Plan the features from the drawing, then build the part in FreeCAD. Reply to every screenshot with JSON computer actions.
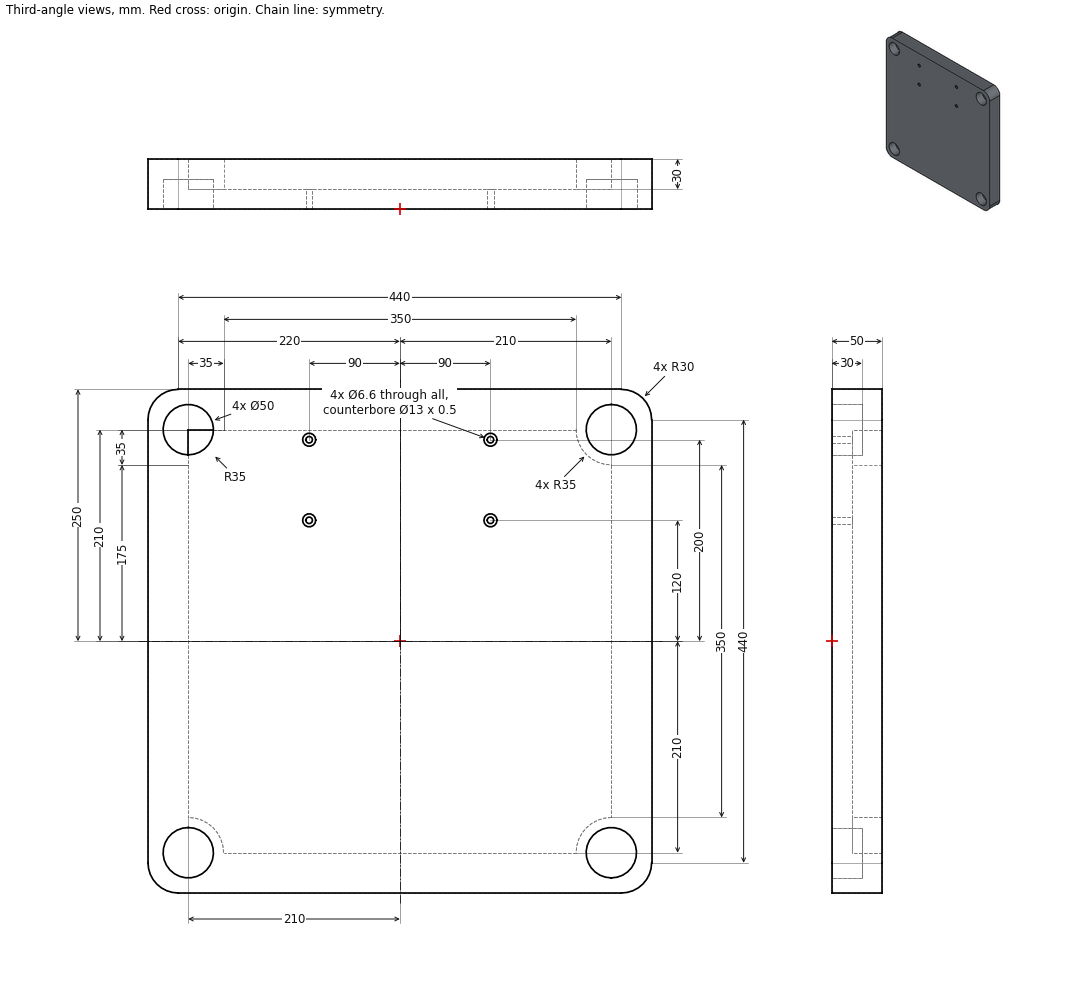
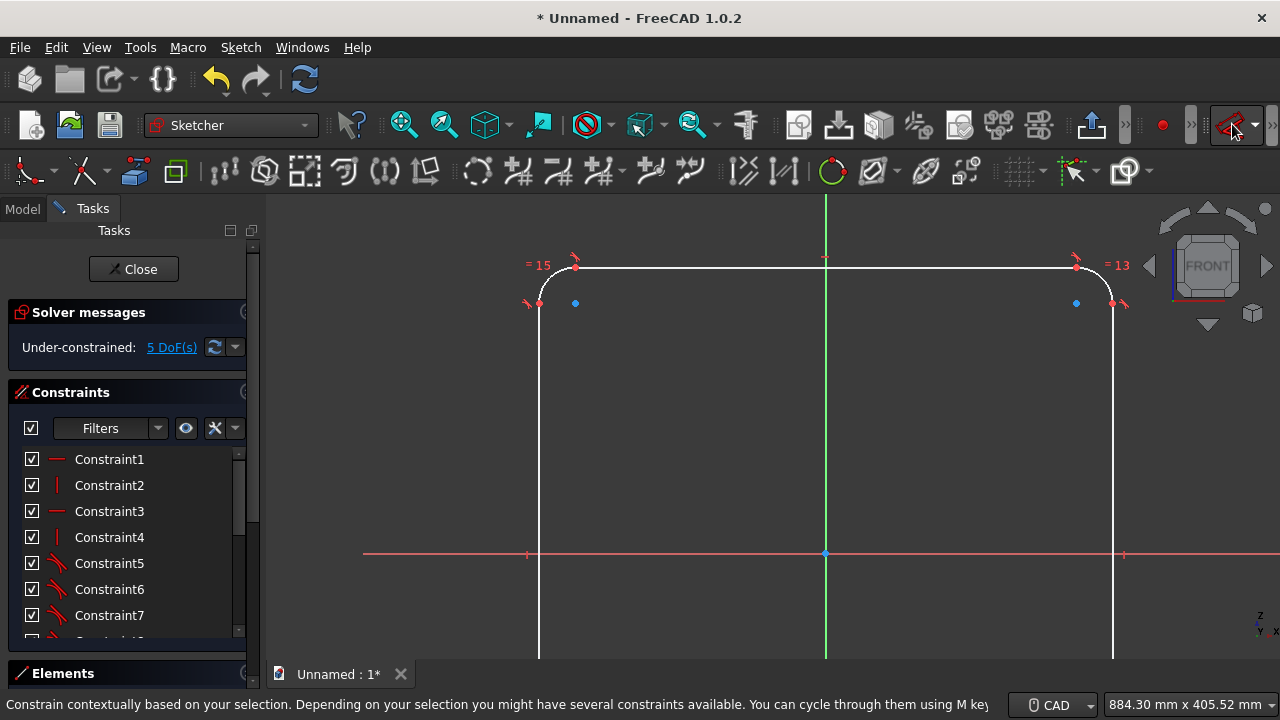
{"action": "left_click", "coordinate": [1109, 287]}
{"action": "left_click", "coordinate": [1083, 235]}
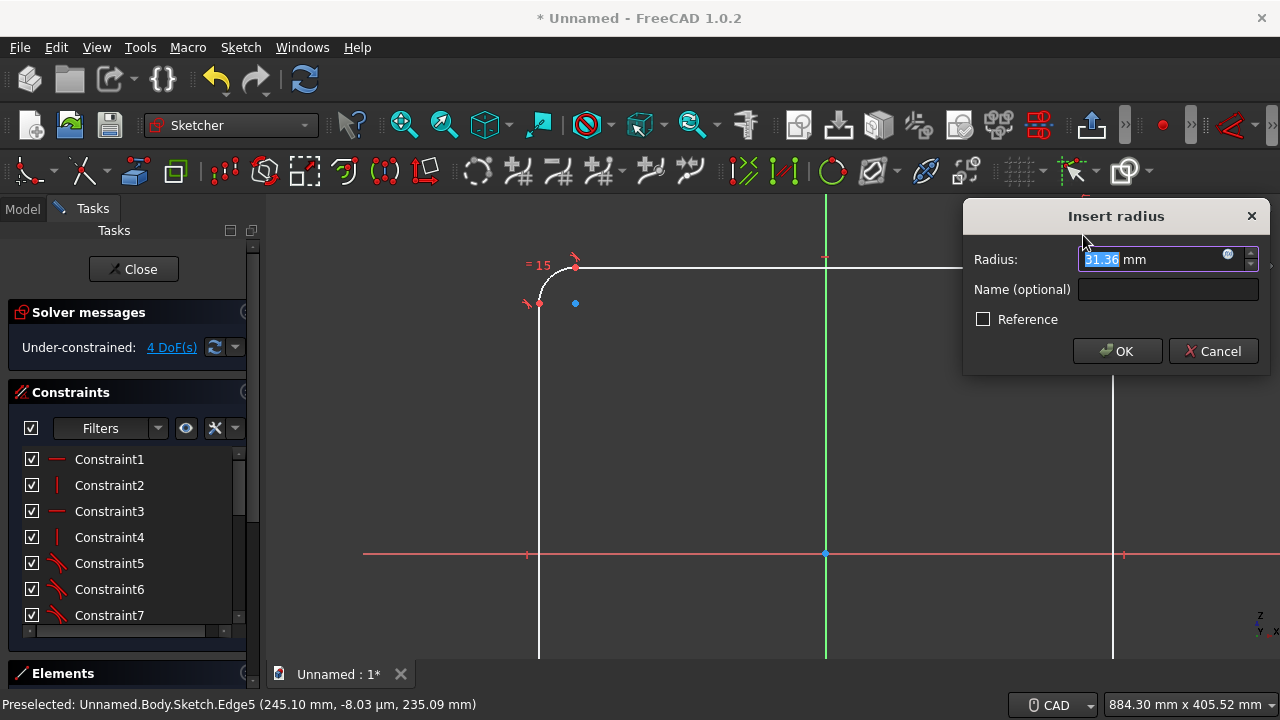
{"action": "type", "text": "30"}
{"action": "key", "text": "Return"}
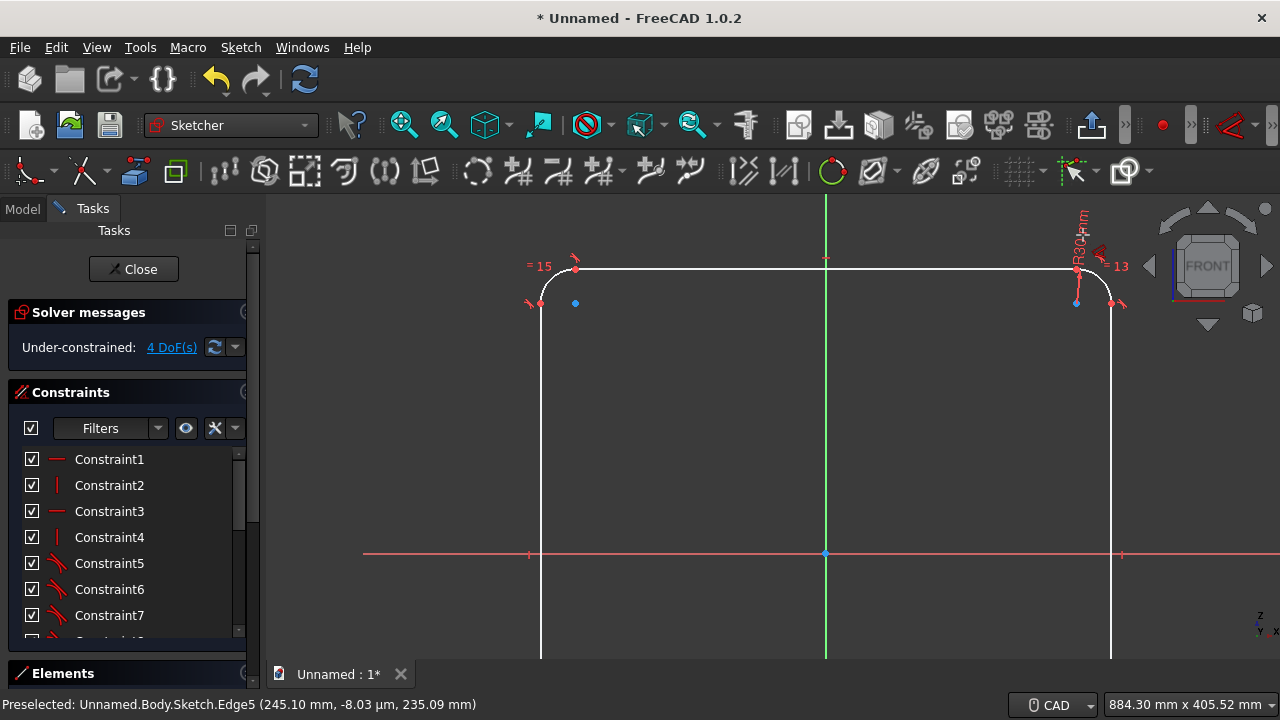
{"action": "left_click", "coordinate": [726, 269]}
{"action": "left_click", "coordinate": [711, 235]}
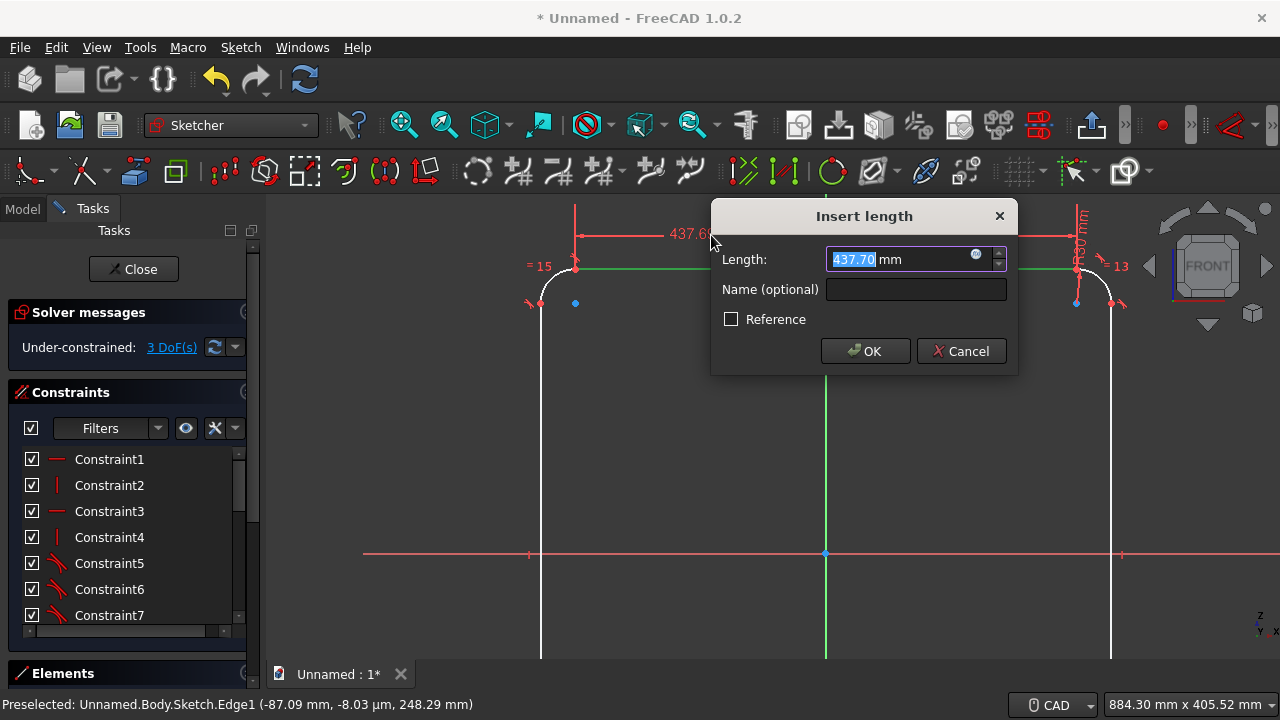
{"action": "type", "text": "440"}
{"action": "key", "text": "Return"}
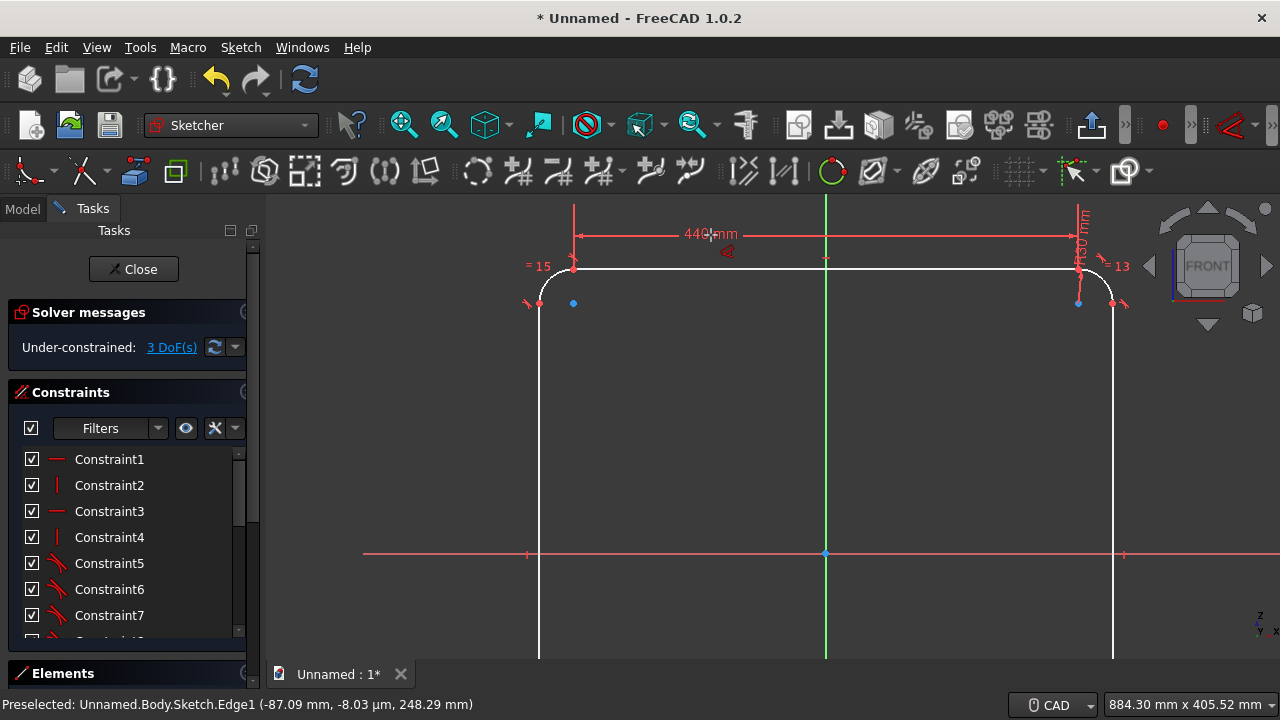
{"action": "left_click", "coordinate": [1113, 454]}
{"action": "left_click", "coordinate": [1079, 467]}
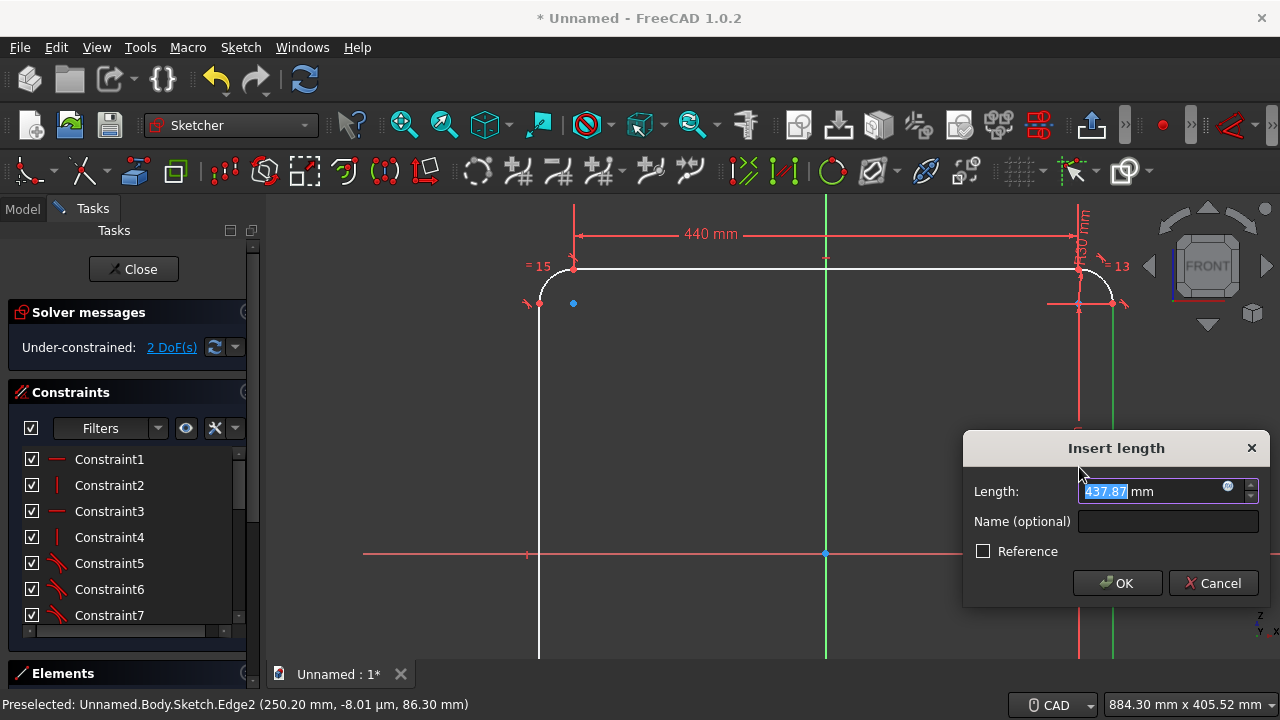
{"action": "type", "text": "440"}
{"action": "key", "text": "Return"}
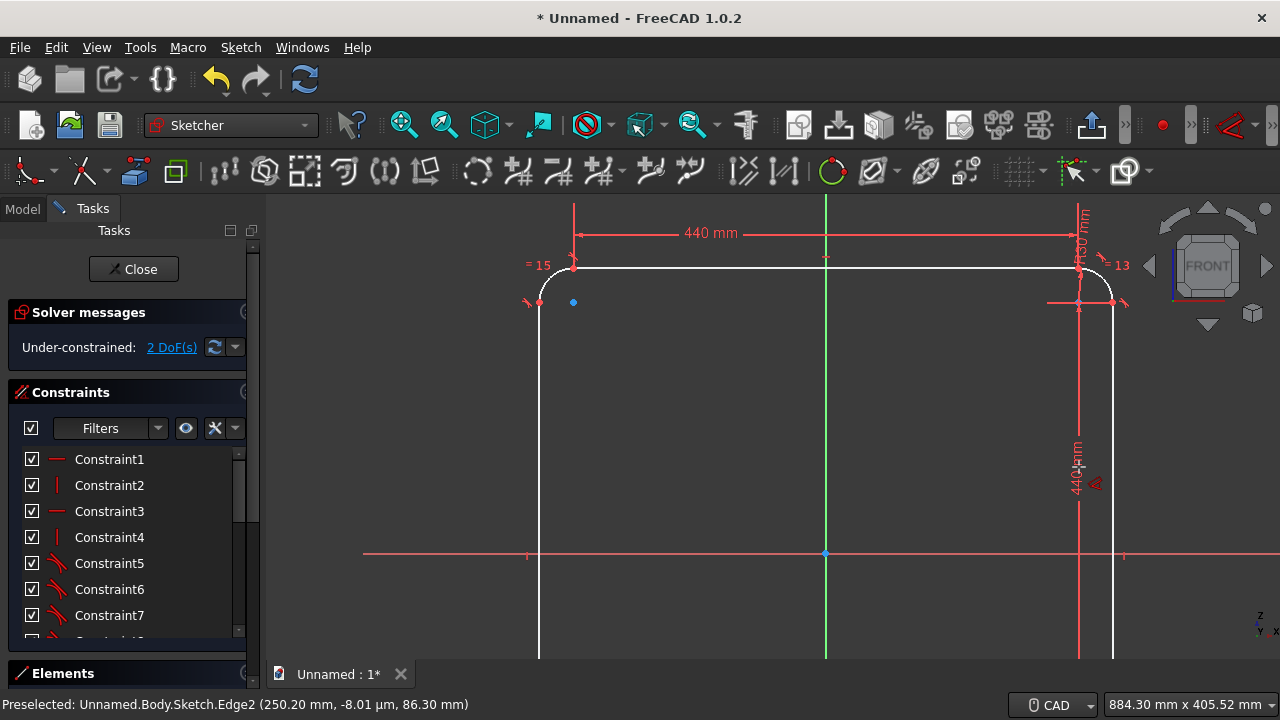
{"action": "left_click", "coordinate": [574, 268]}
{"action": "left_click", "coordinate": [612, 234]}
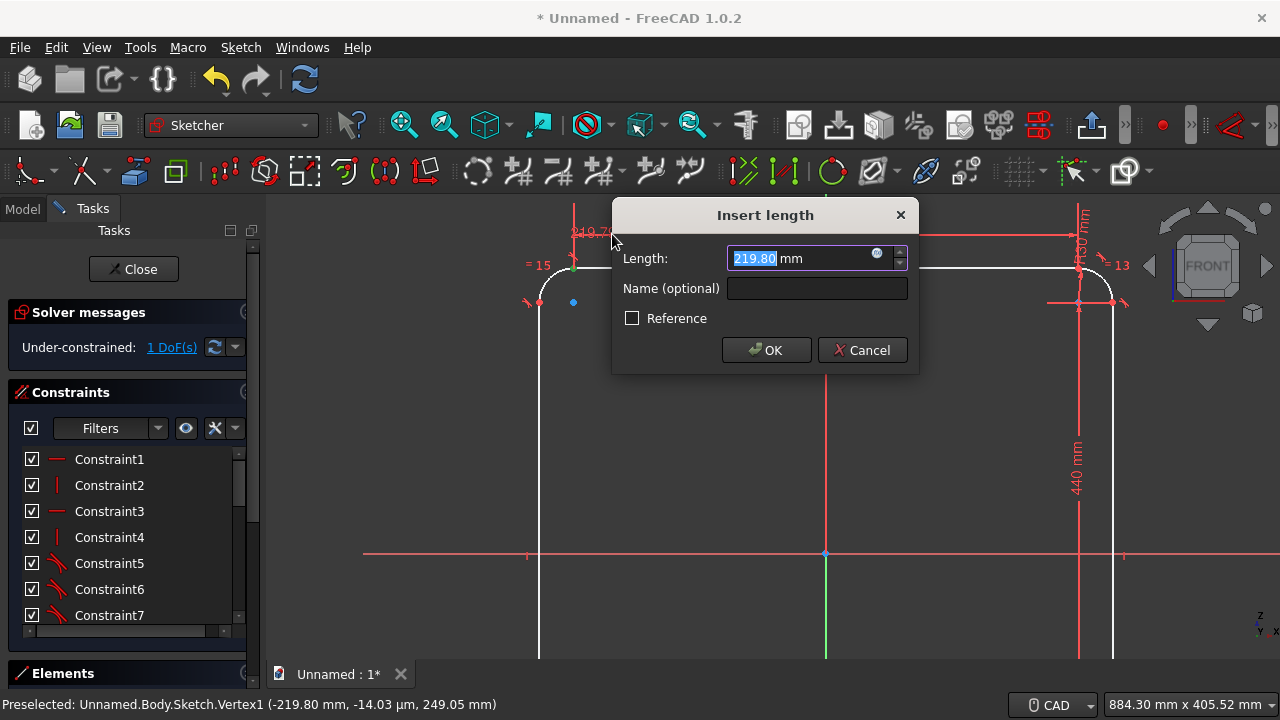
{"action": "type", "text": "220"}
{"action": "key", "text": "Return"}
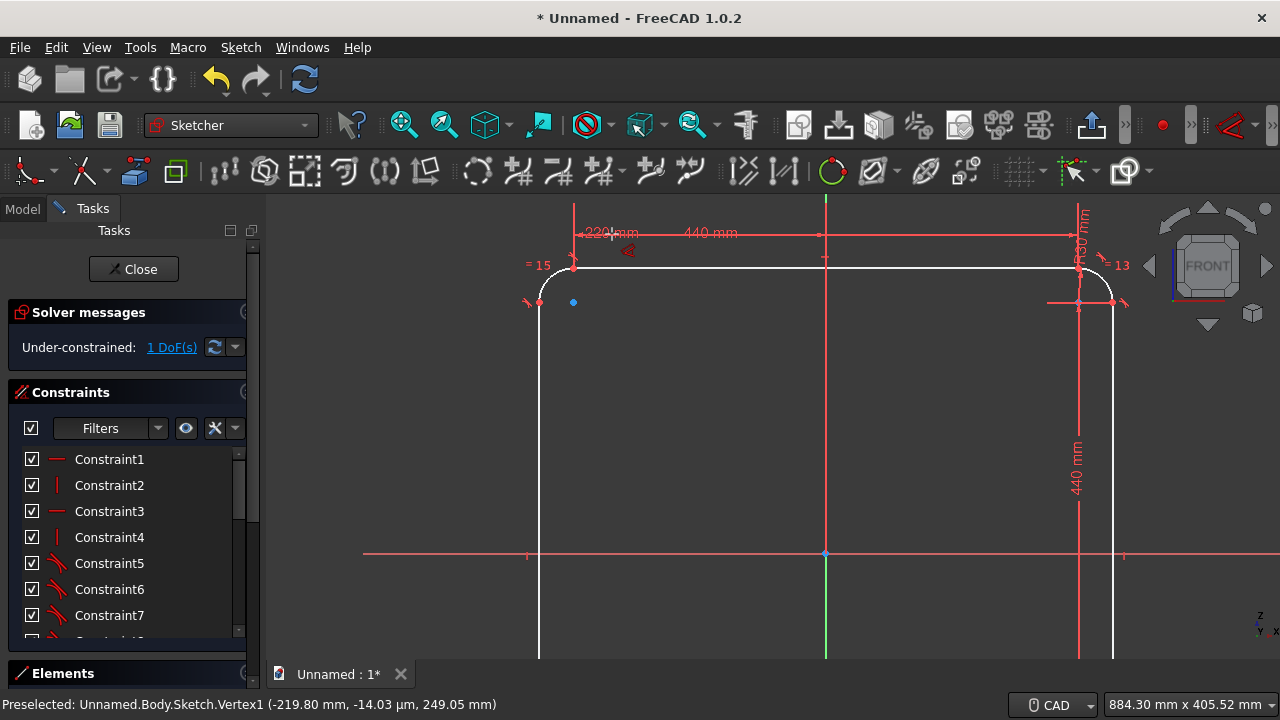
{"action": "left_click", "coordinate": [574, 268]}
{"action": "left_click", "coordinate": [860, 411]}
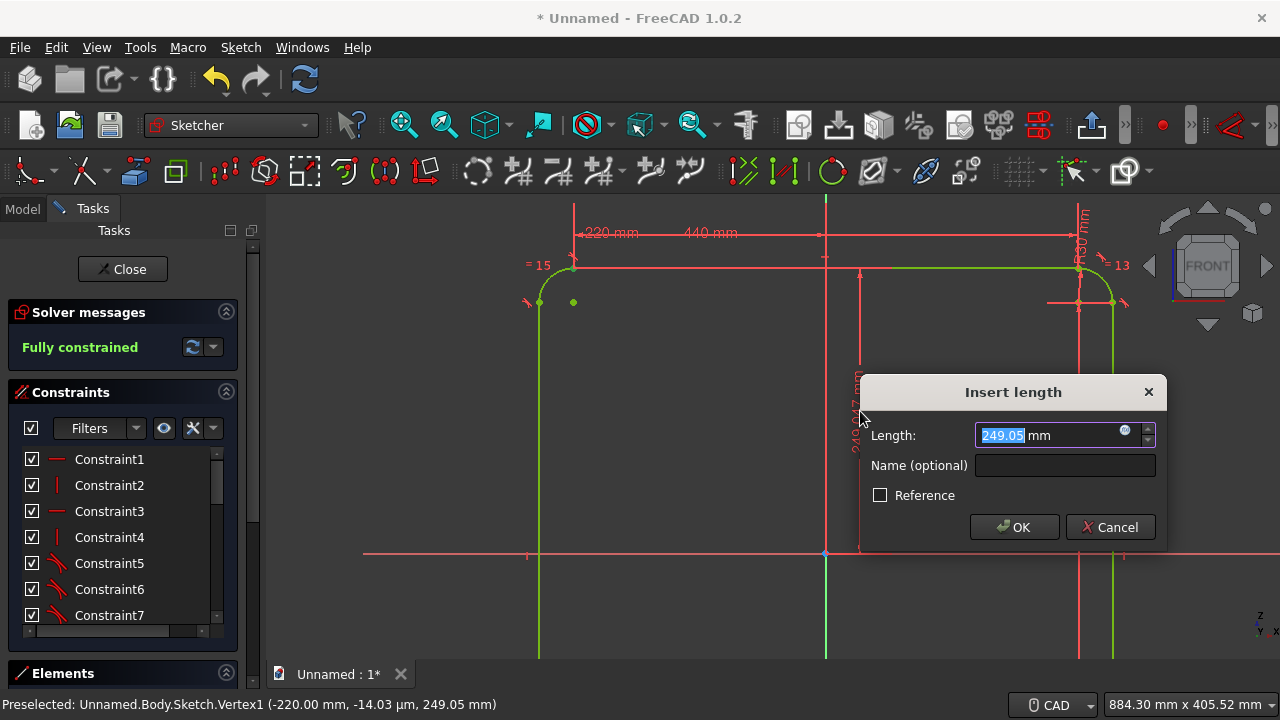
{"action": "type", "text": "250"}
{"action": "key", "text": "Return"}
{"action": "key", "text": "Escape"}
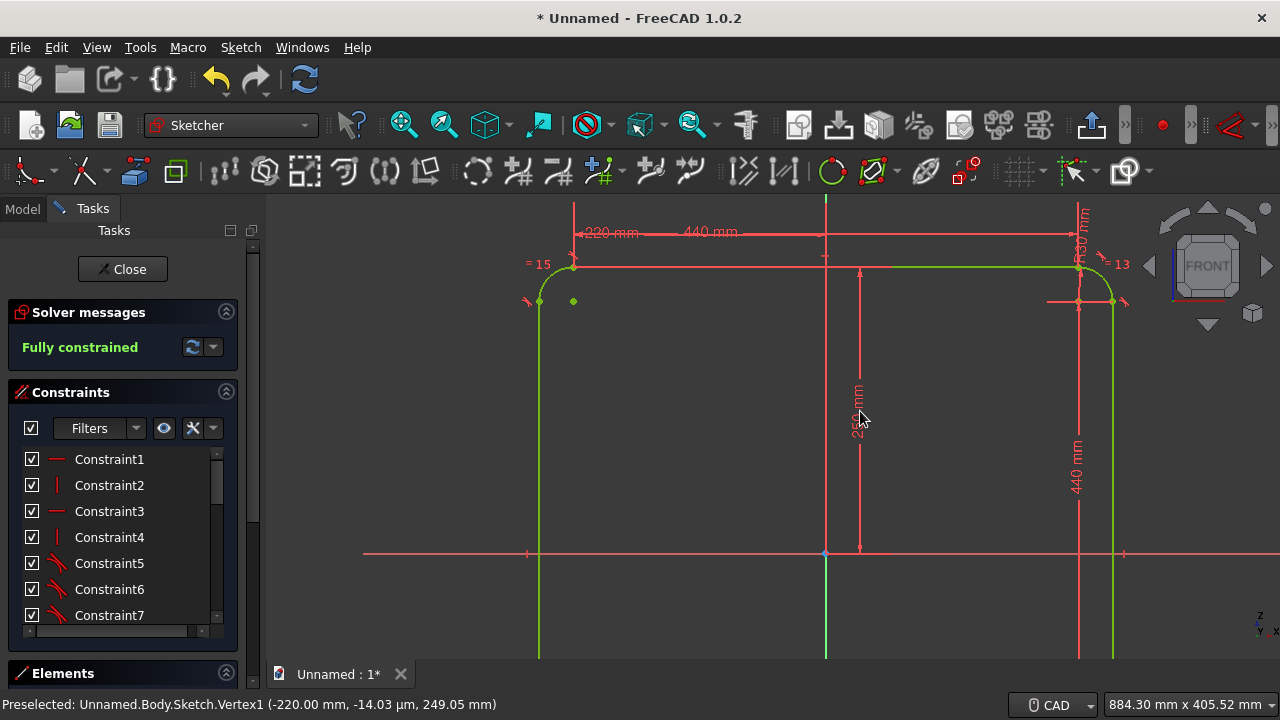
{"action": "left_click", "coordinate": [123, 269]}